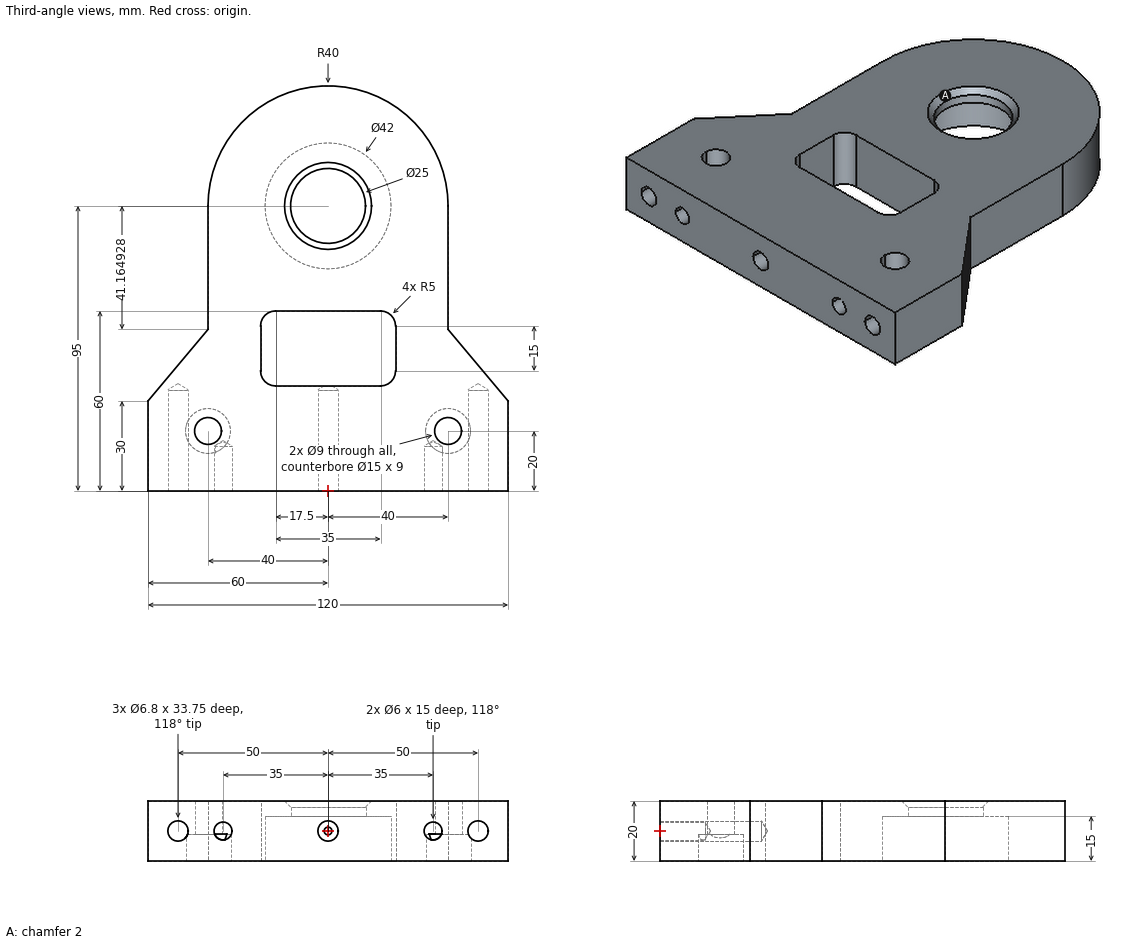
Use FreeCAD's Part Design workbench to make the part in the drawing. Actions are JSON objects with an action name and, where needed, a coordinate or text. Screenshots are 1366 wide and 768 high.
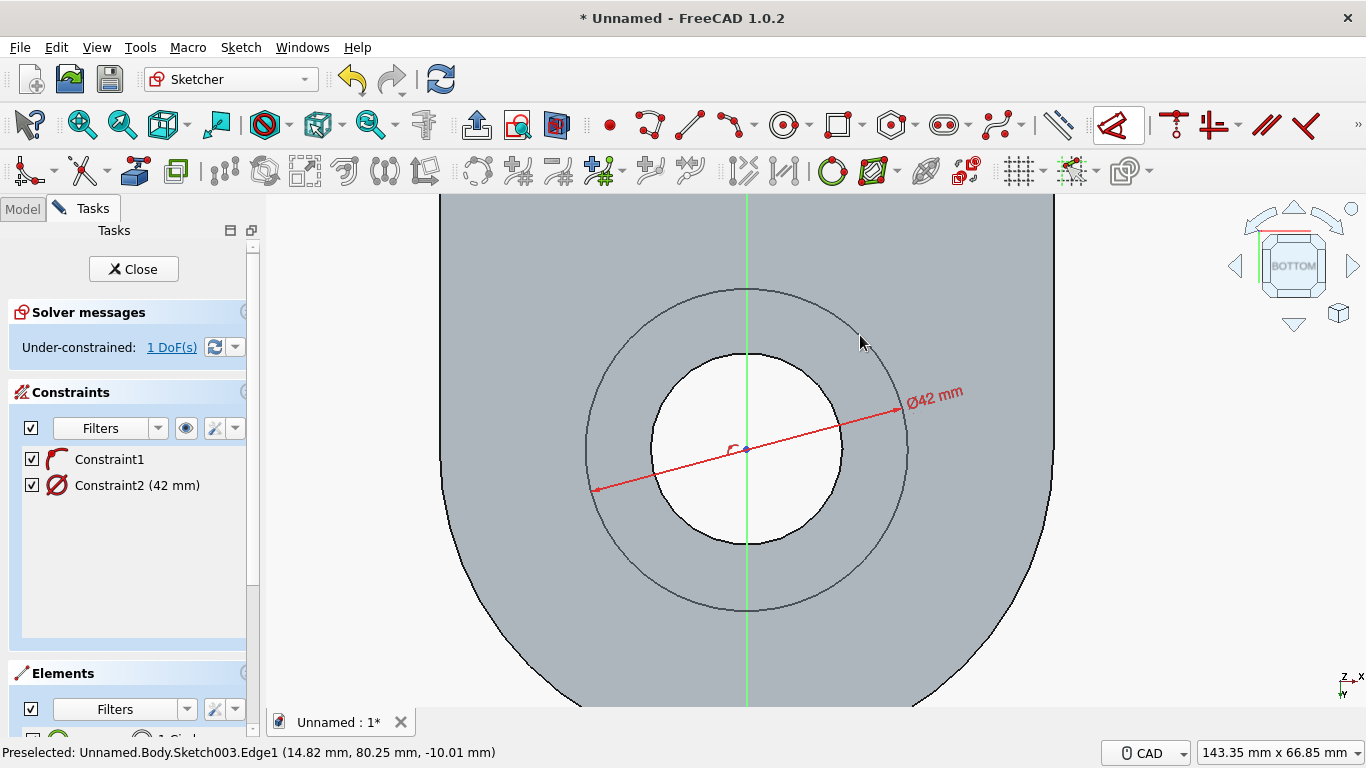
{"action": "left_click", "coordinate": [747, 450]}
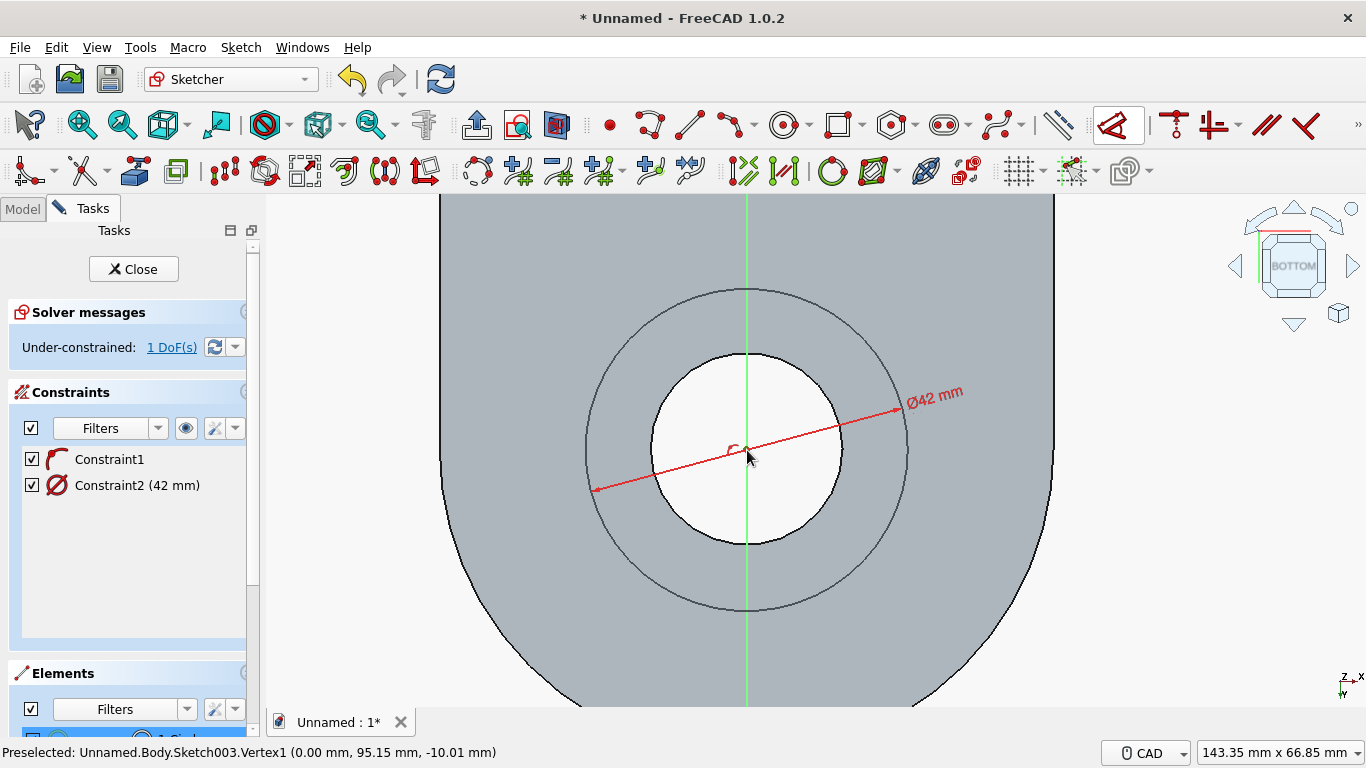
{"action": "left_click", "coordinate": [1138, 126]}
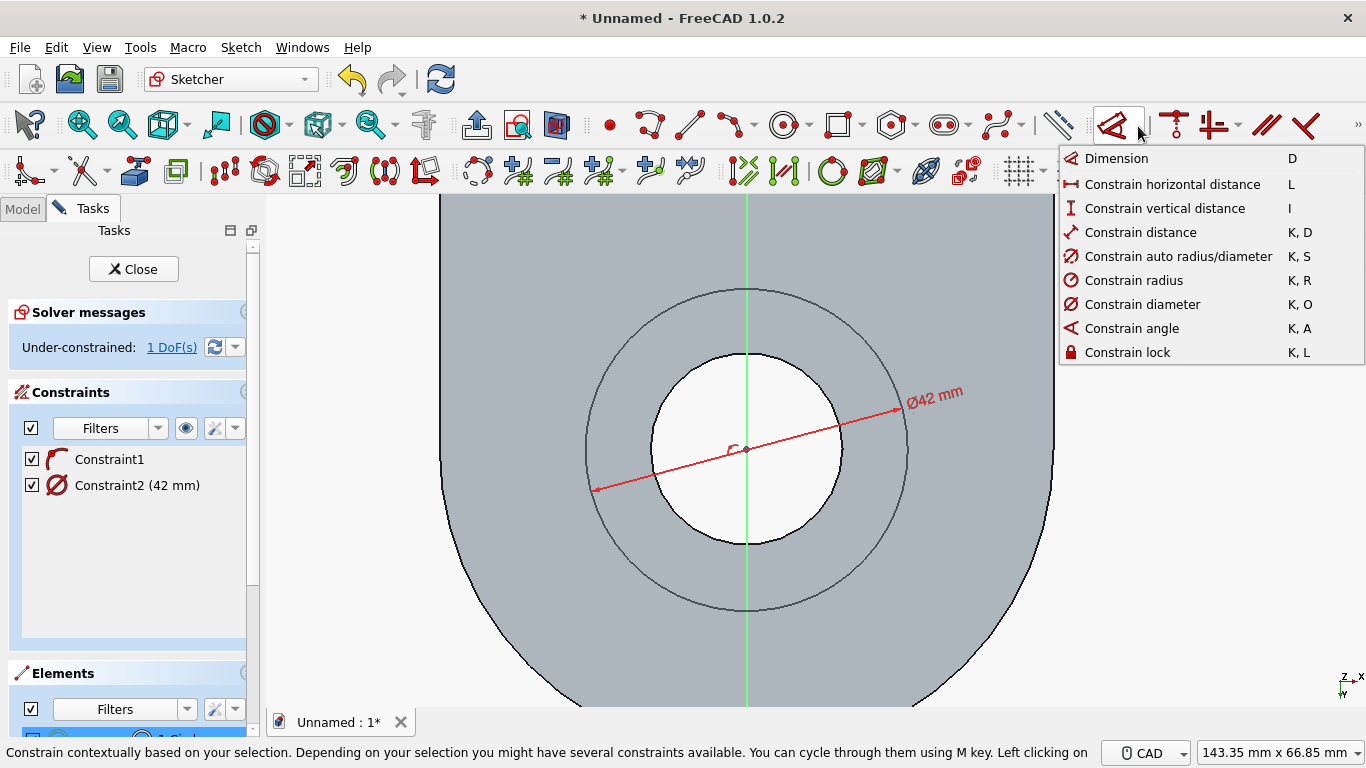
{"action": "left_click", "coordinate": [1212, 208]}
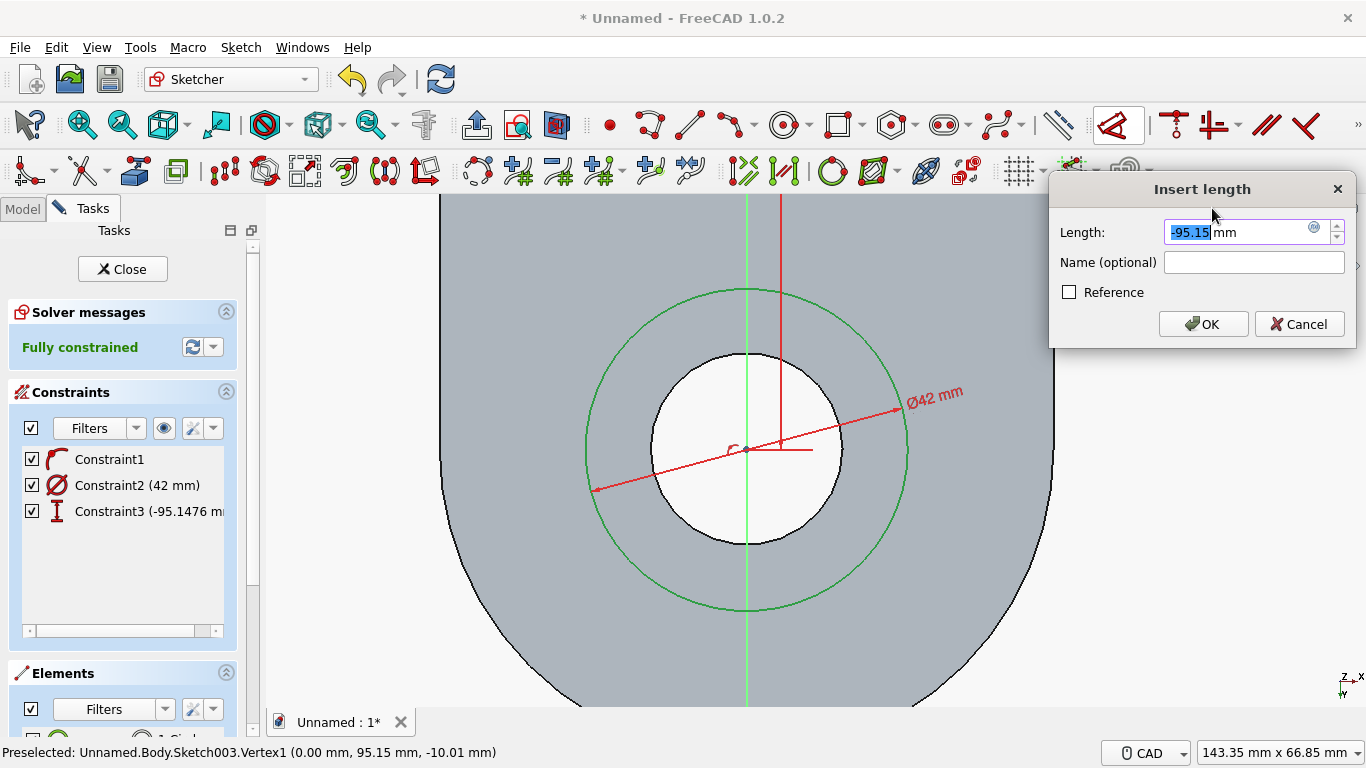
{"action": "type", "text": "-95"}
{"action": "key", "text": "Return"}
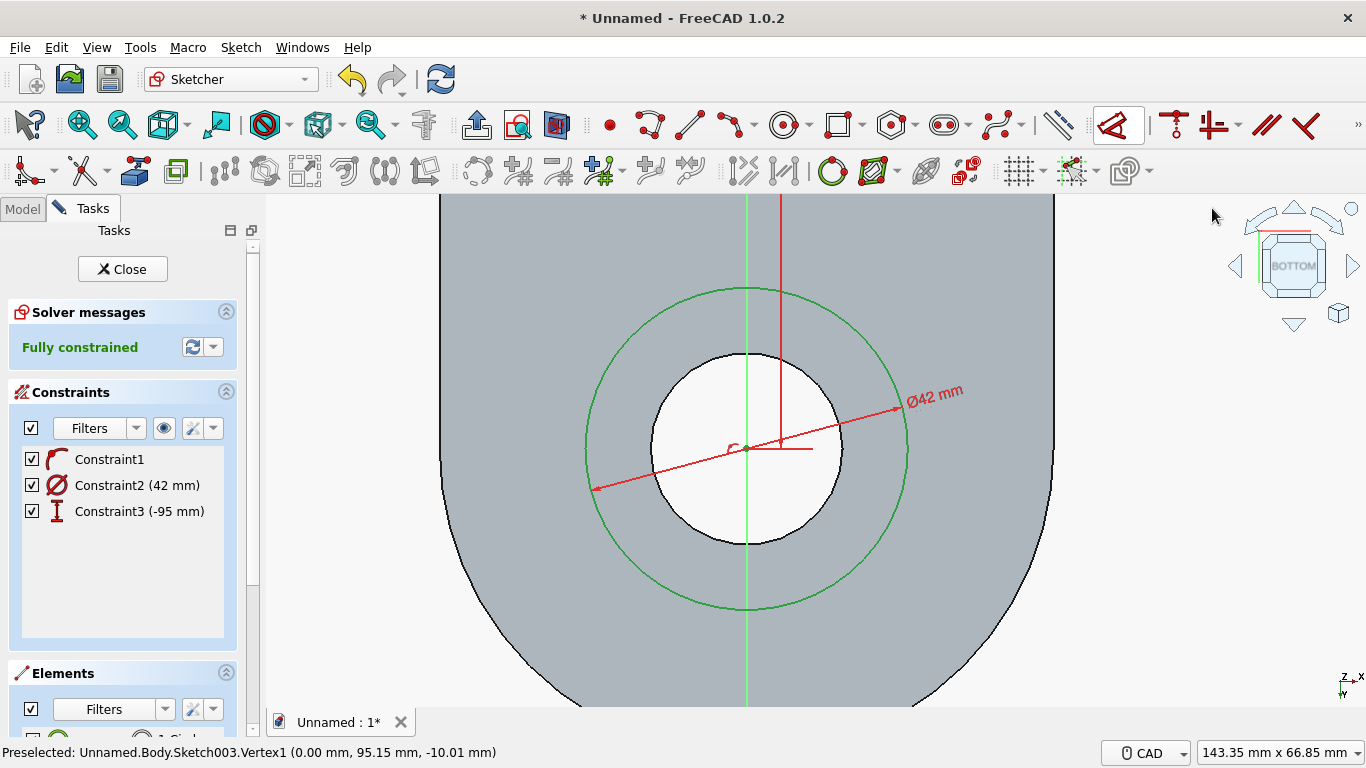
{"action": "left_click", "coordinate": [123, 269]}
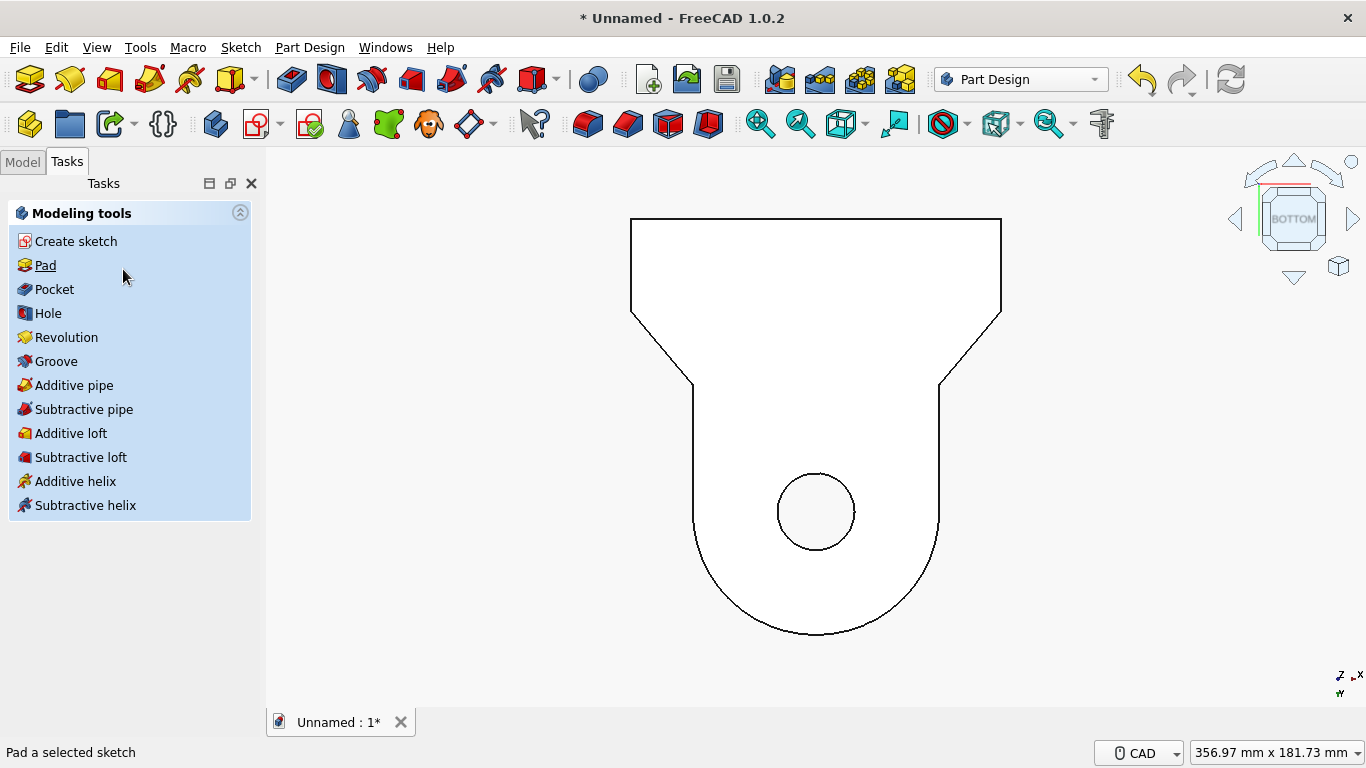
{"action": "left_click", "coordinate": [292, 80]}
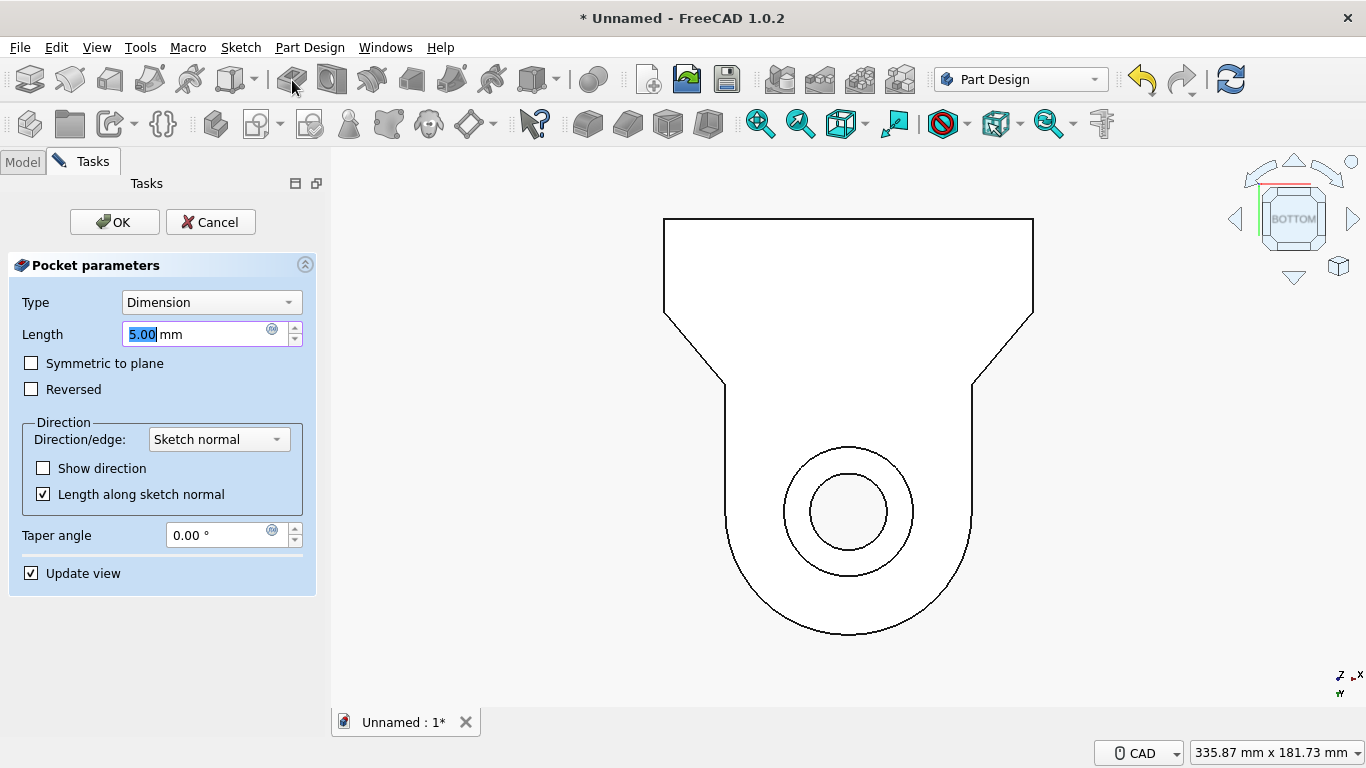
{"action": "type", "text": "15"}
{"action": "key", "text": "Tab"}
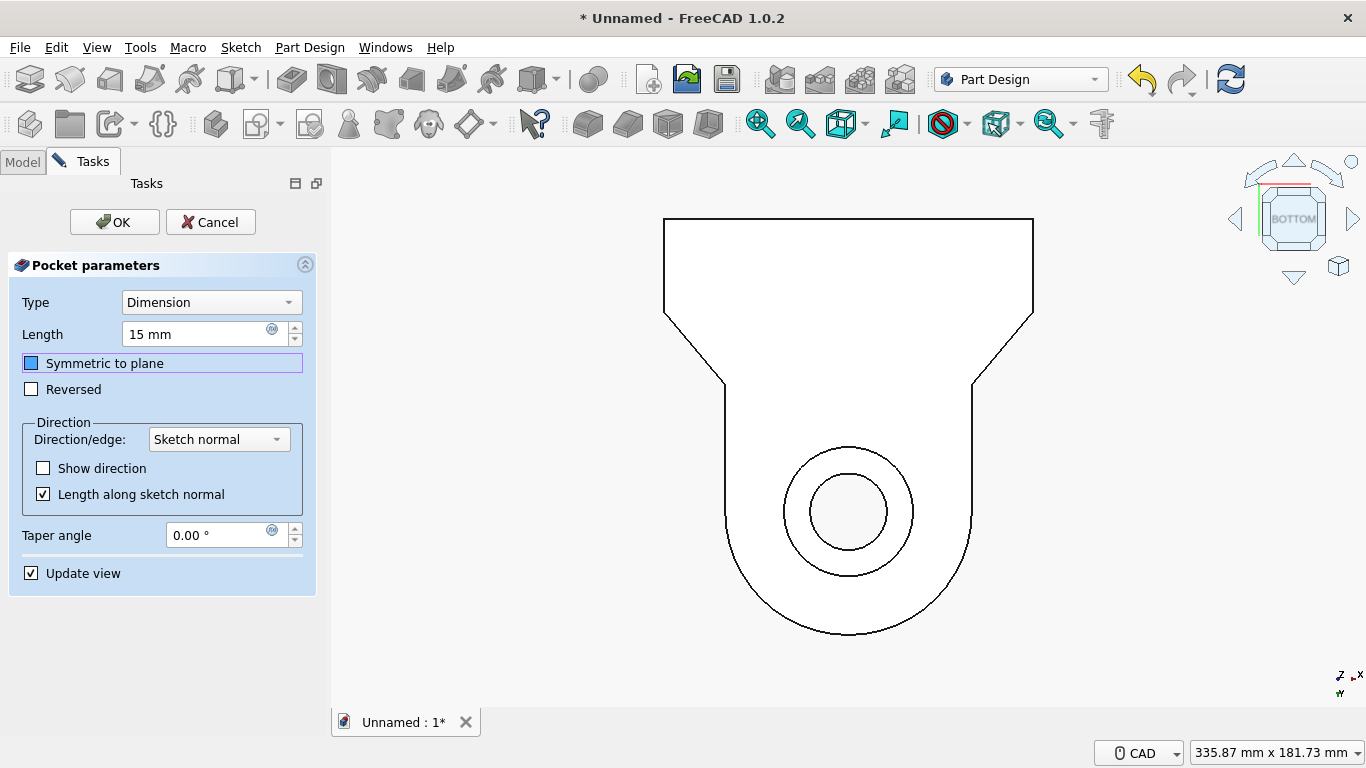
{"action": "left_click", "coordinate": [115, 222]}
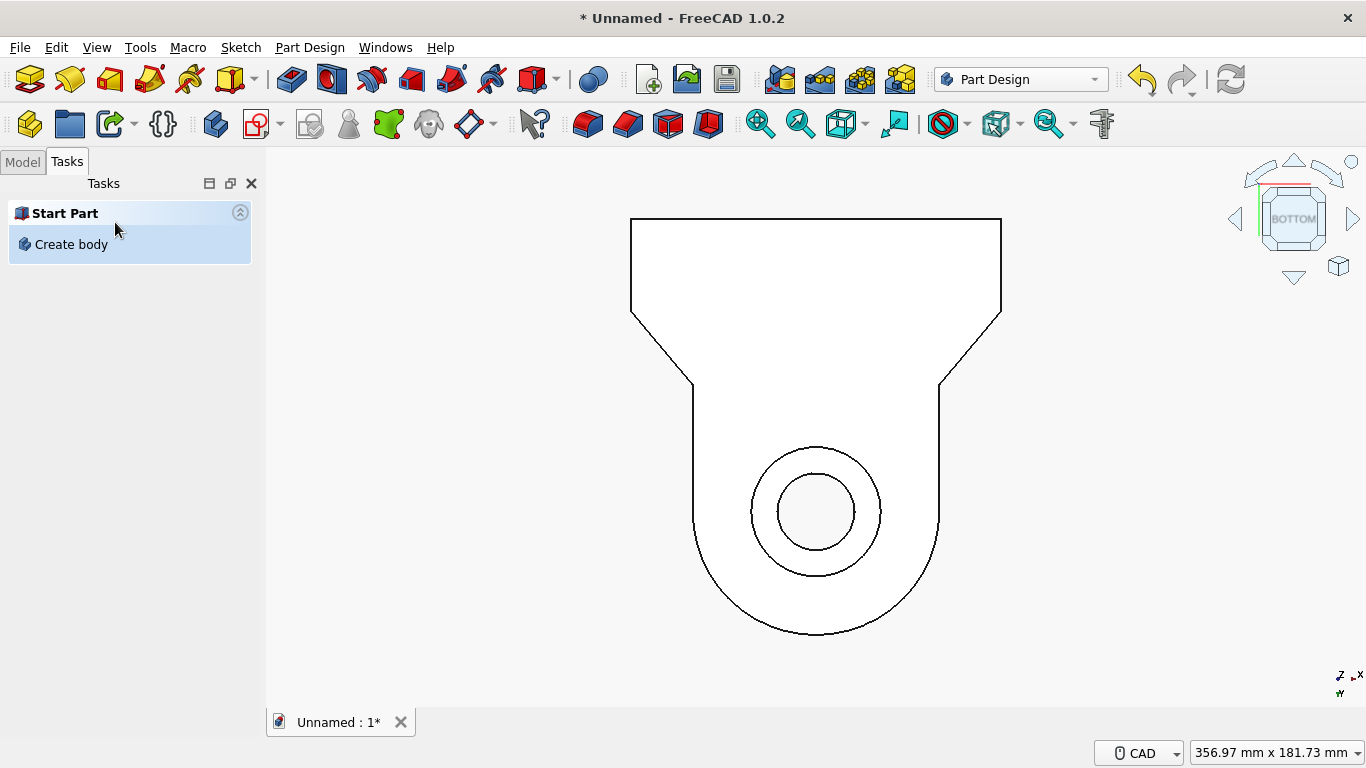
{"action": "key", "text": "0"}